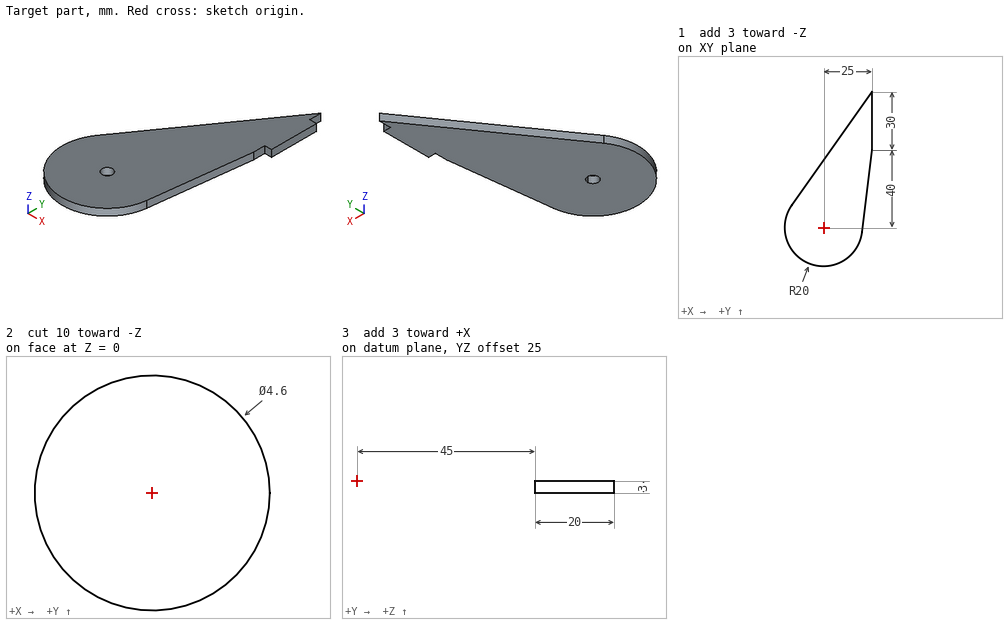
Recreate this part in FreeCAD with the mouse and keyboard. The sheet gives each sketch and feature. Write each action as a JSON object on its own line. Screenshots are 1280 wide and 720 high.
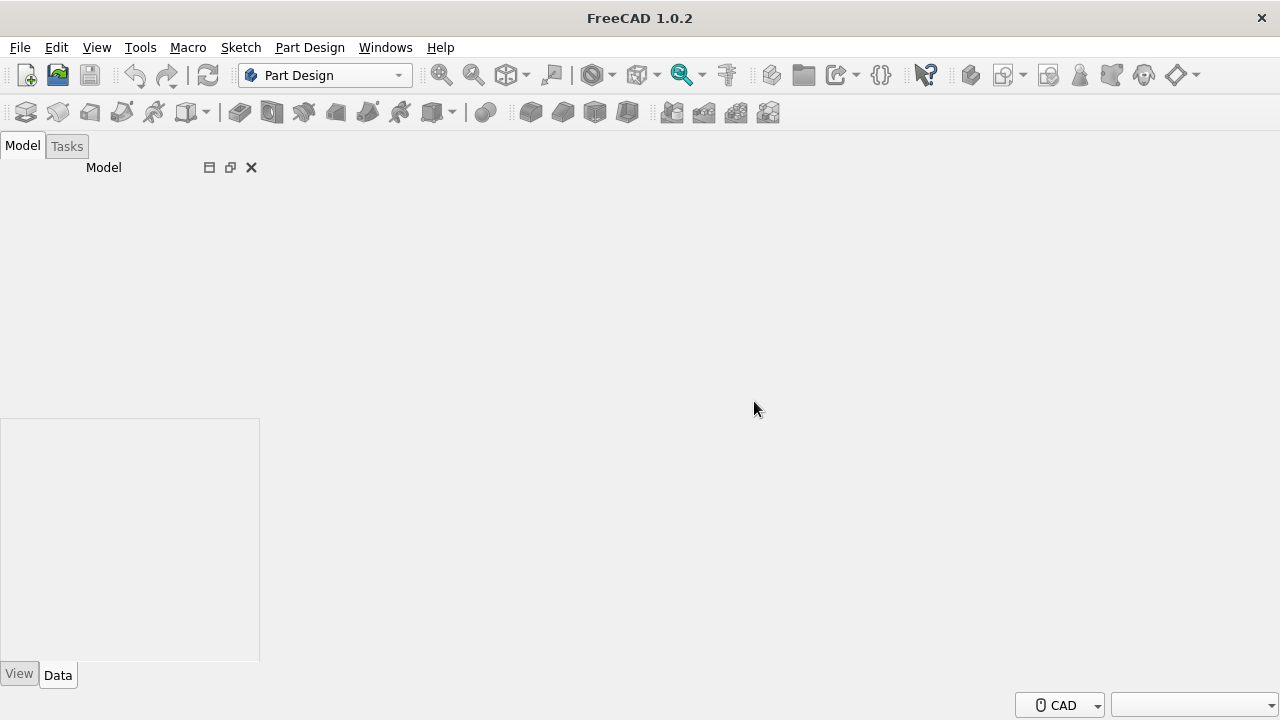
{"action": "left_click", "coordinate": [26, 76]}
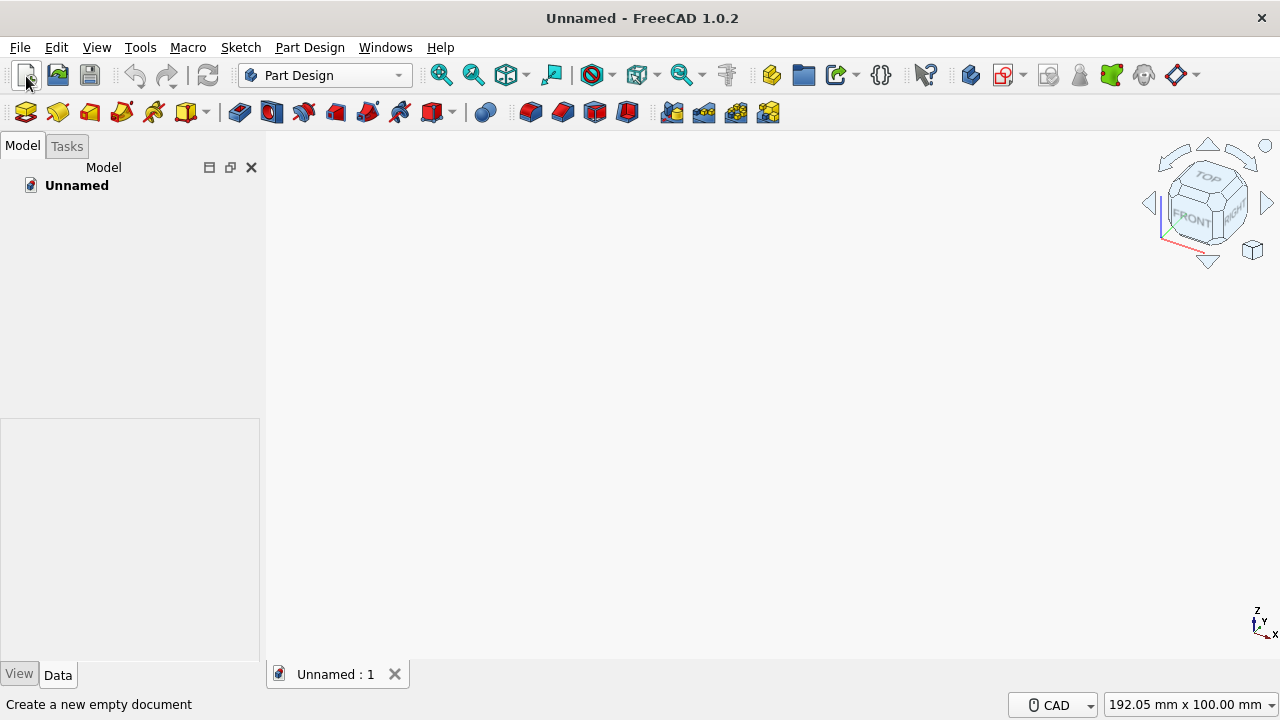
{"action": "left_click", "coordinate": [1004, 76]}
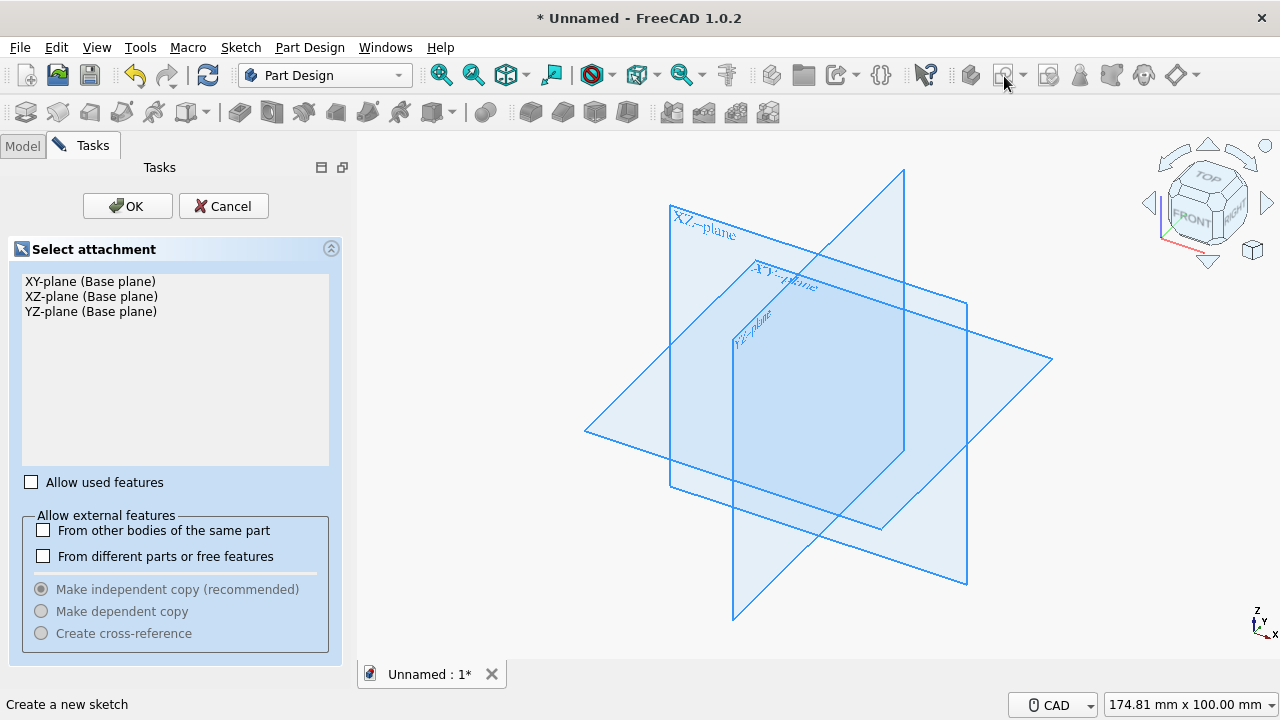
{"action": "left_click", "coordinate": [82, 282]}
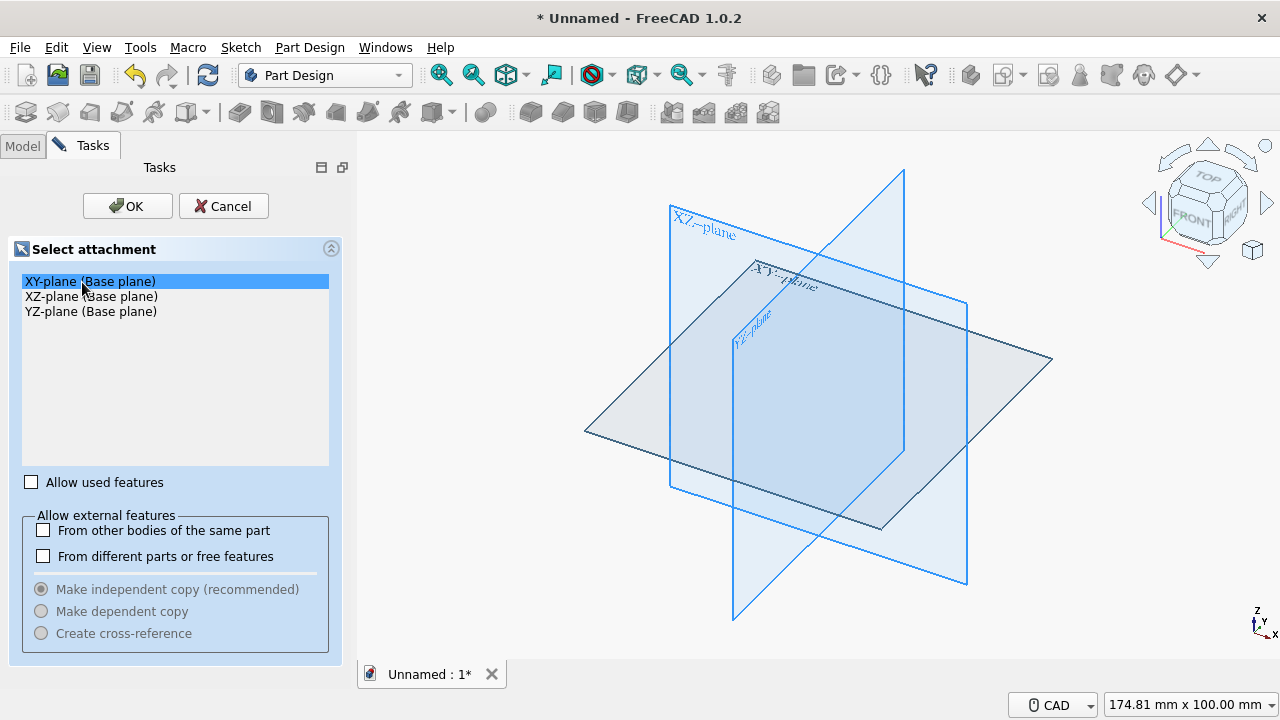
{"action": "left_click", "coordinate": [128, 206]}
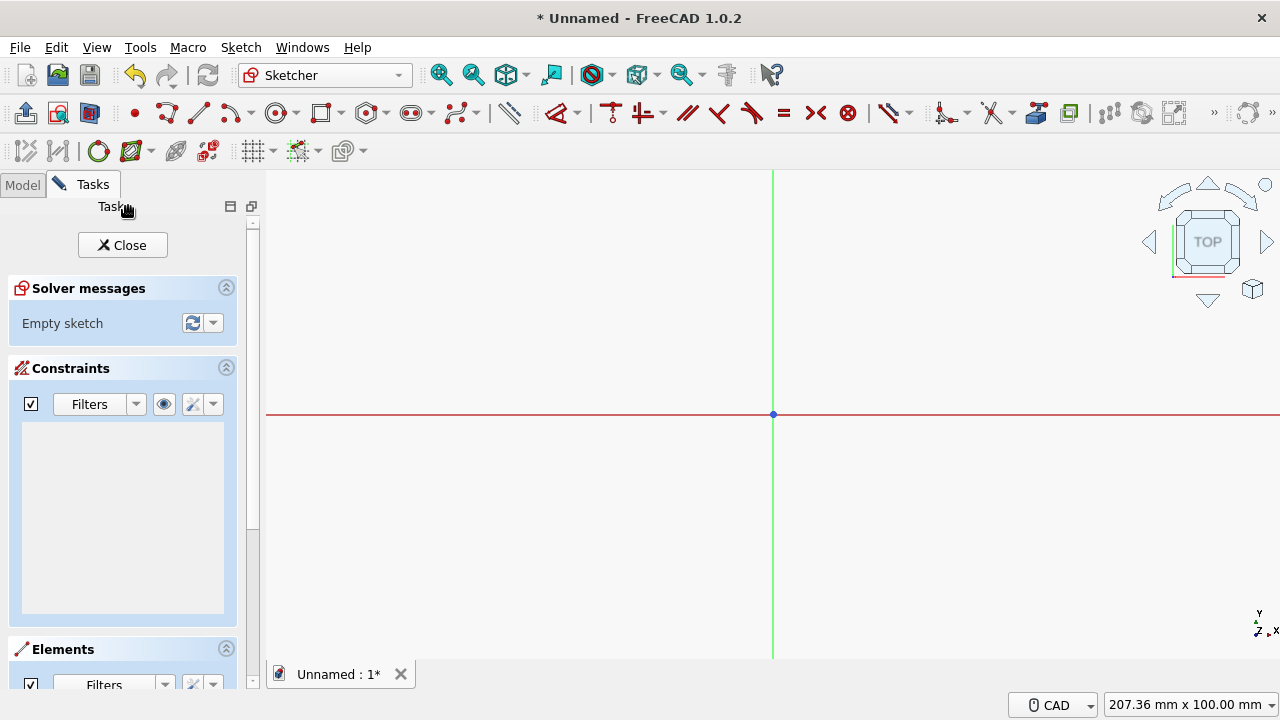
{"action": "scroll", "coordinate": [522, 631], "scroll_direction": "down", "scroll_amount": 2}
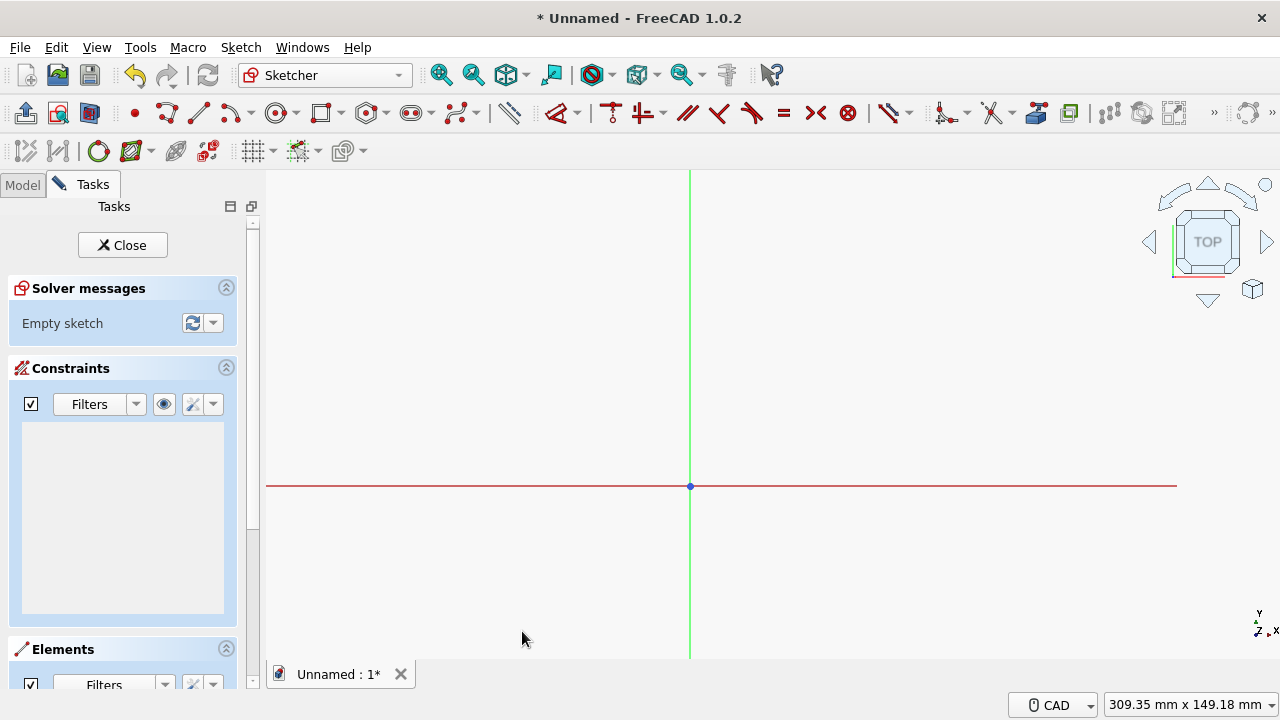
{"action": "left_click", "coordinate": [168, 114]}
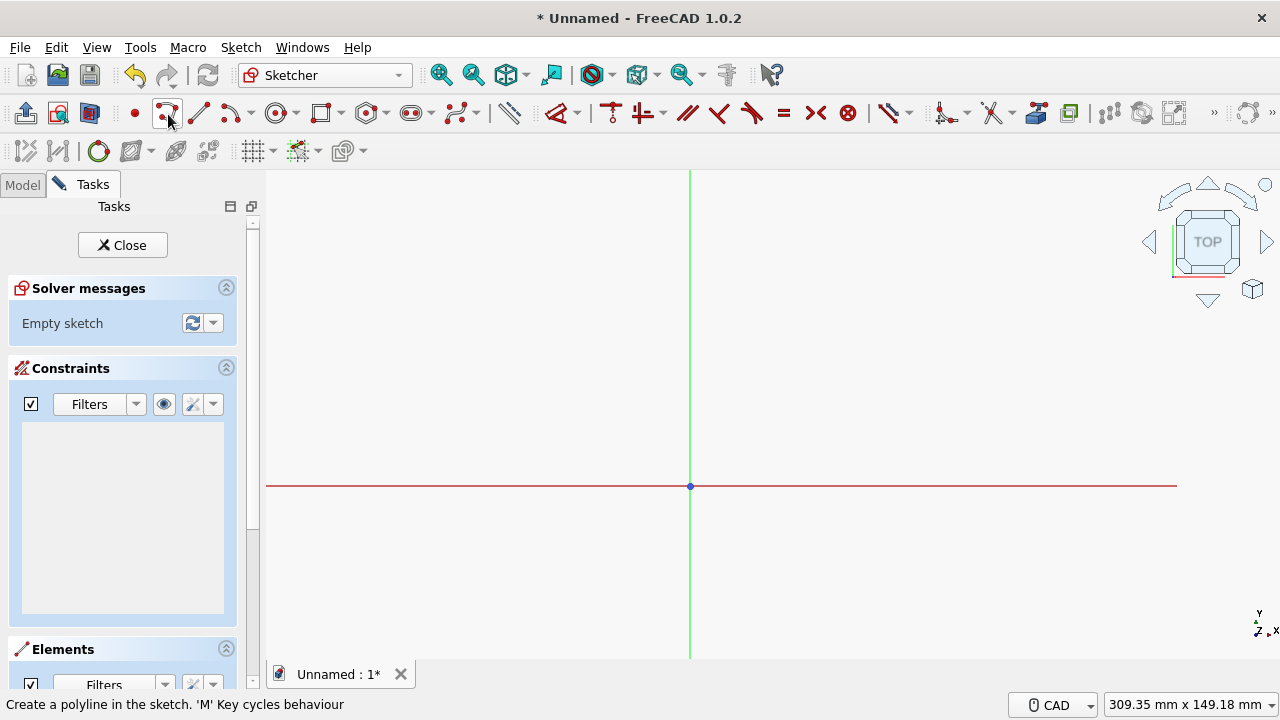
{"action": "scroll", "coordinate": [755, 494], "scroll_direction": "up", "scroll_amount": 4}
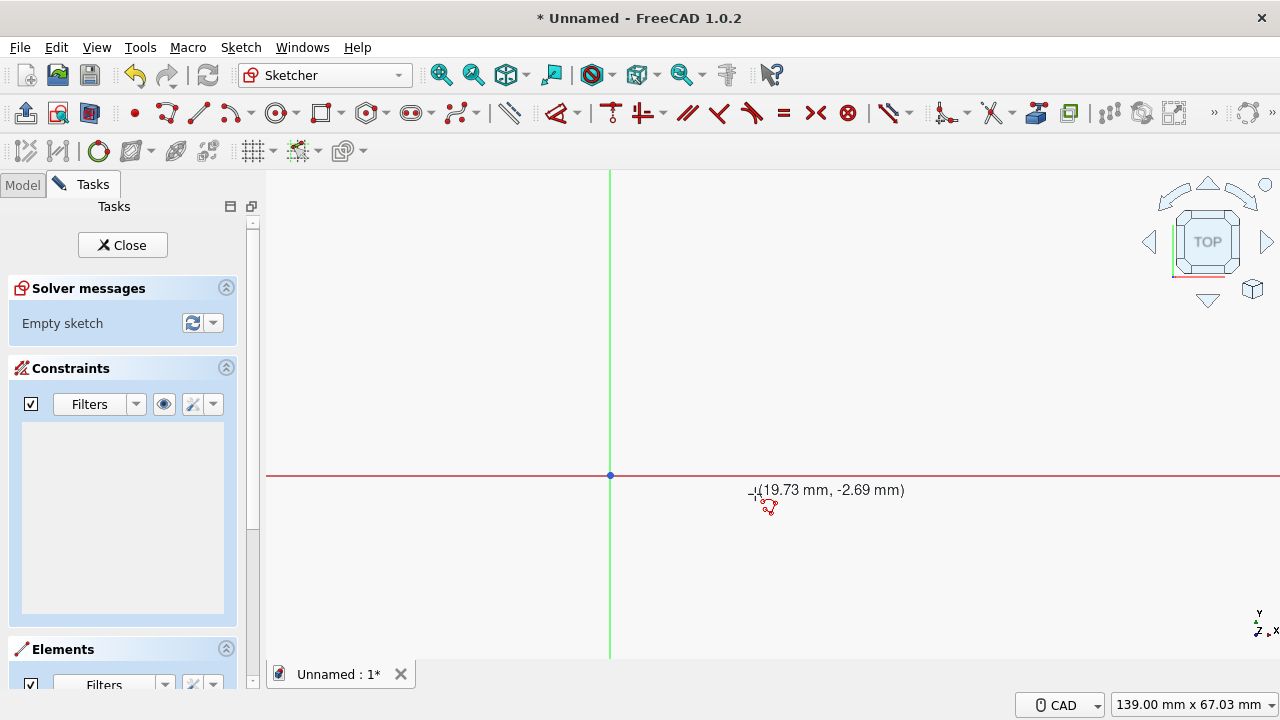
{"action": "left_click", "coordinate": [755, 493]}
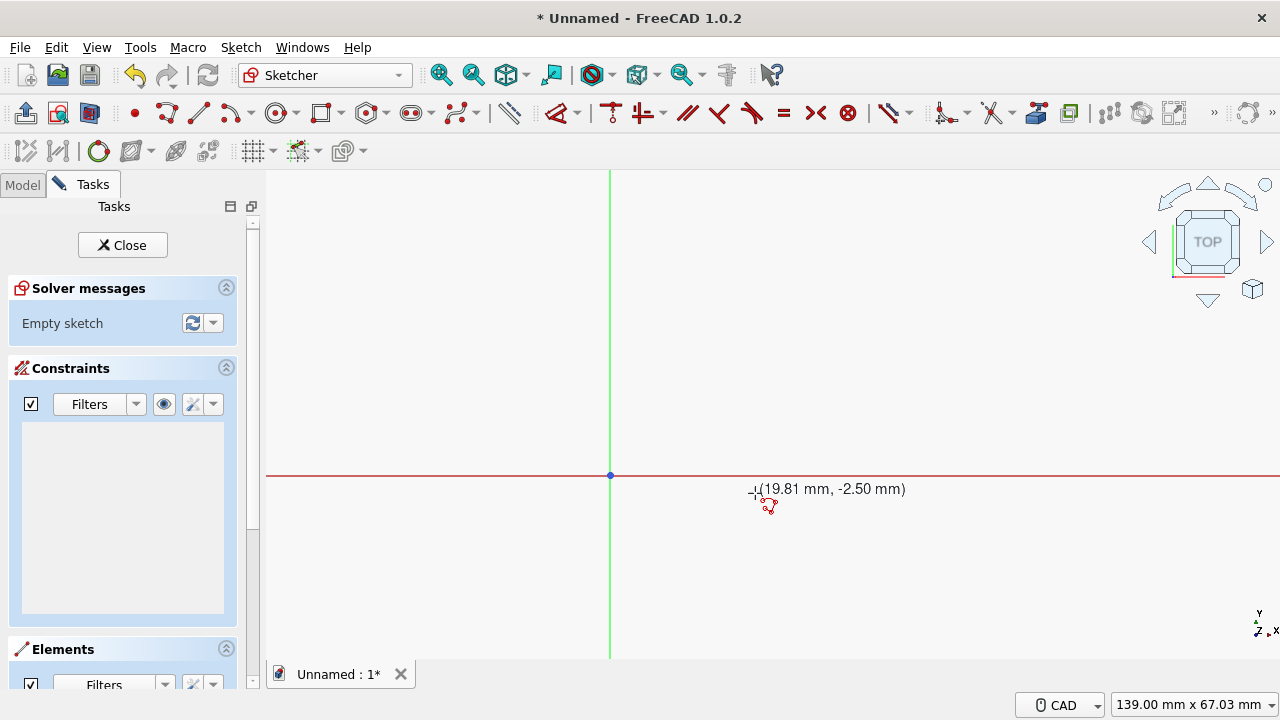
{"action": "scroll", "coordinate": [755, 517], "scroll_direction": "down", "scroll_amount": 4}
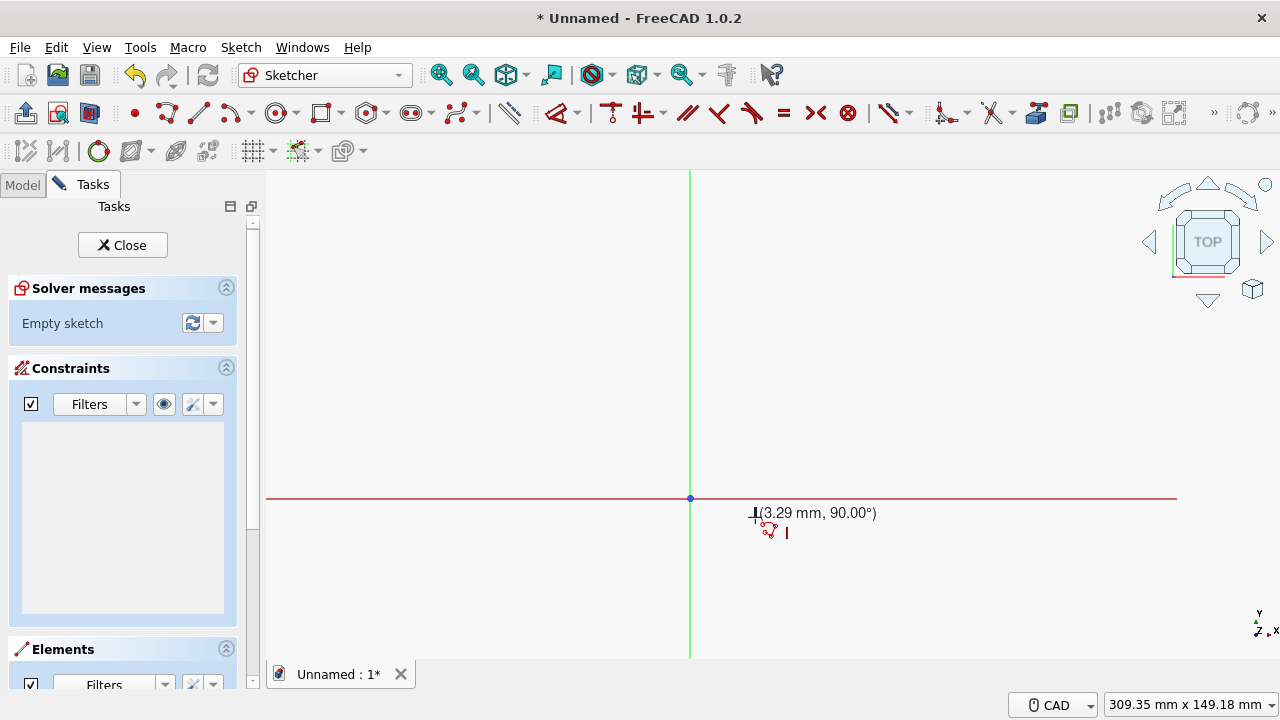
{"action": "left_click", "coordinate": [772, 368]}
{"action": "left_click", "coordinate": [772, 269]}
{"action": "left_click", "coordinate": [637, 461]}
{"action": "right_click", "coordinate": [637, 461]}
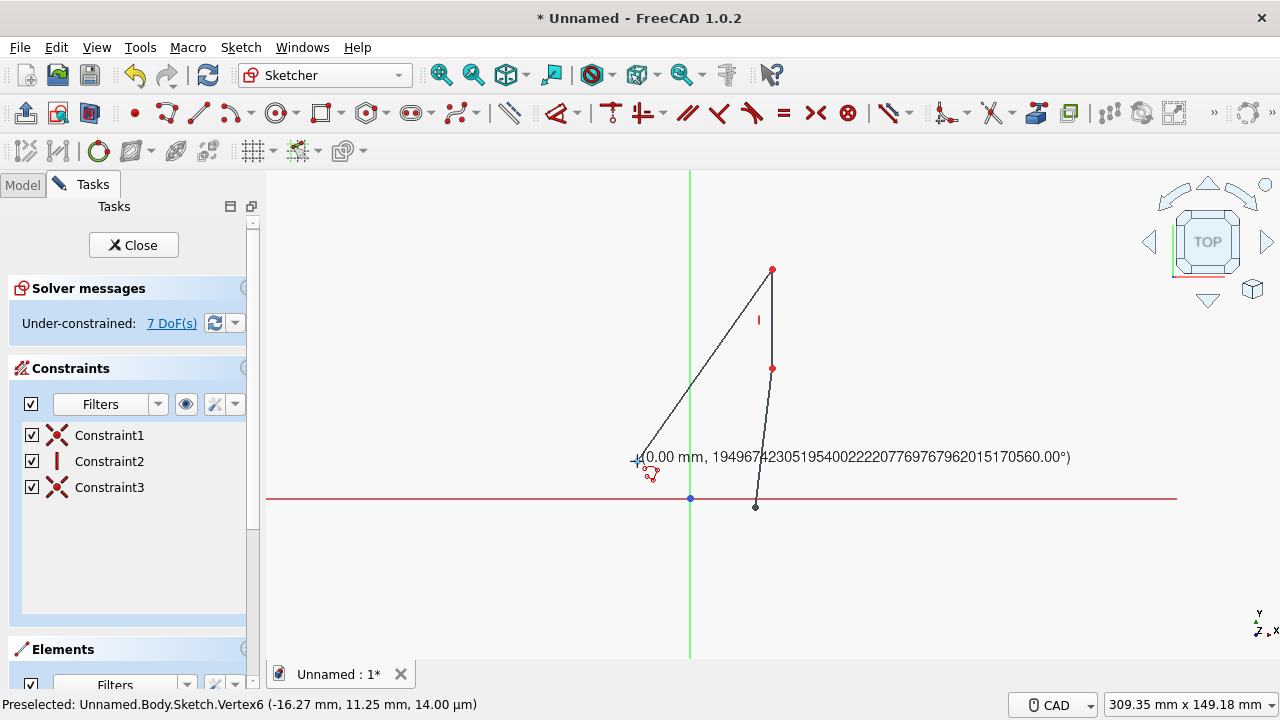
{"action": "key", "text": "g 3 a"}